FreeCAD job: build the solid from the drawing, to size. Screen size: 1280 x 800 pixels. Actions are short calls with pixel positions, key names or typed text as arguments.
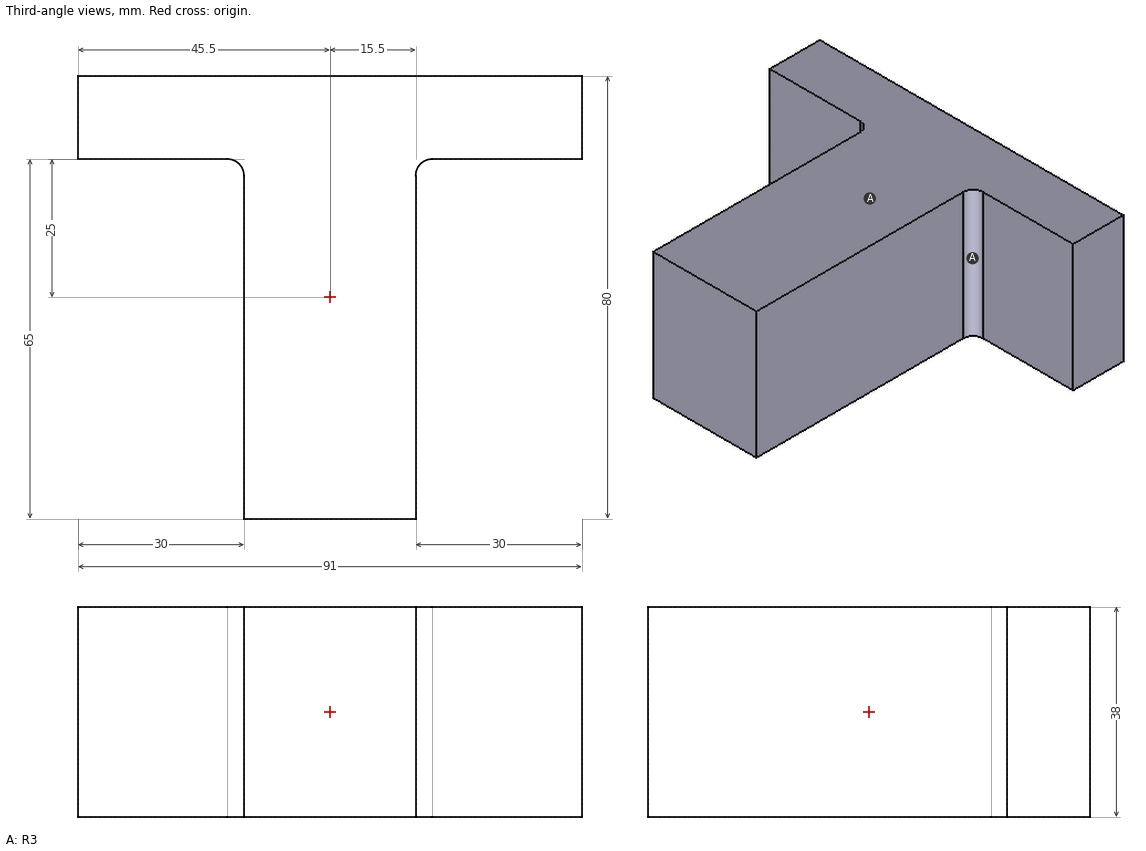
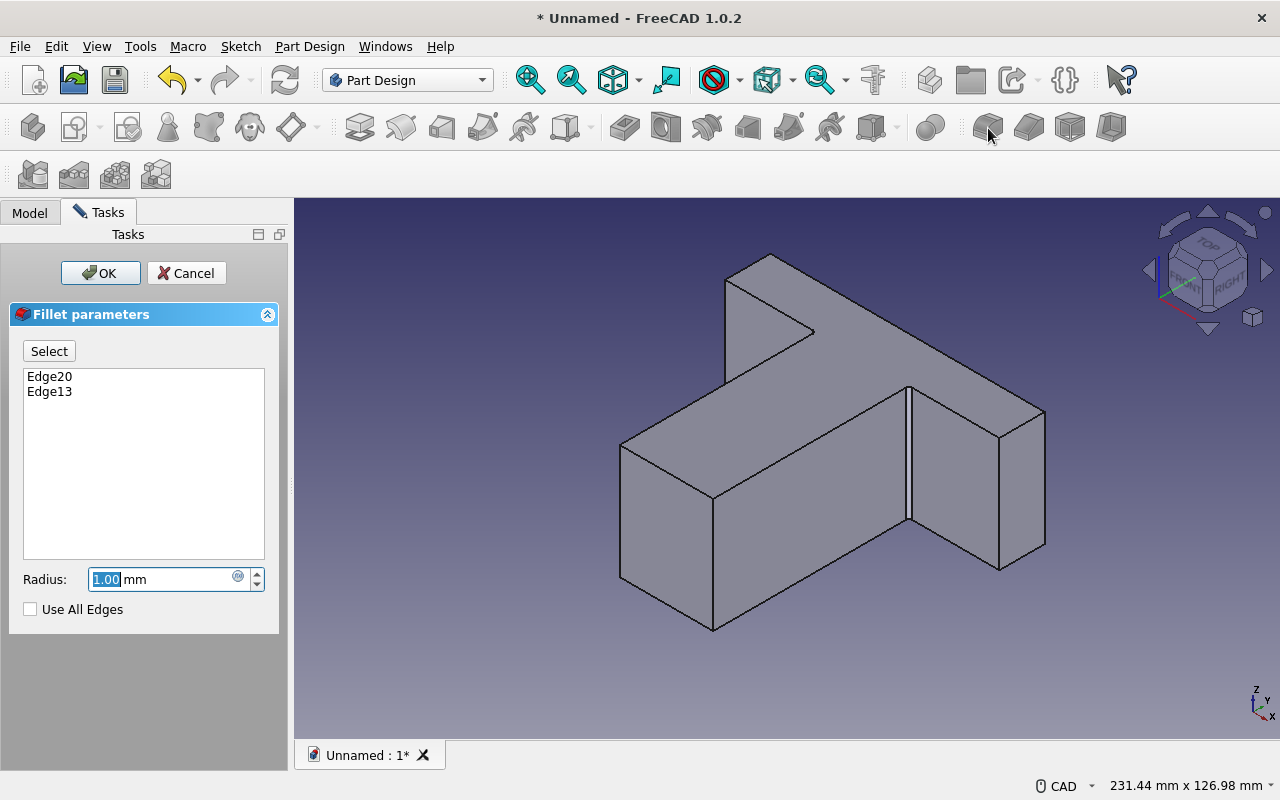
text(3)
key(Tab)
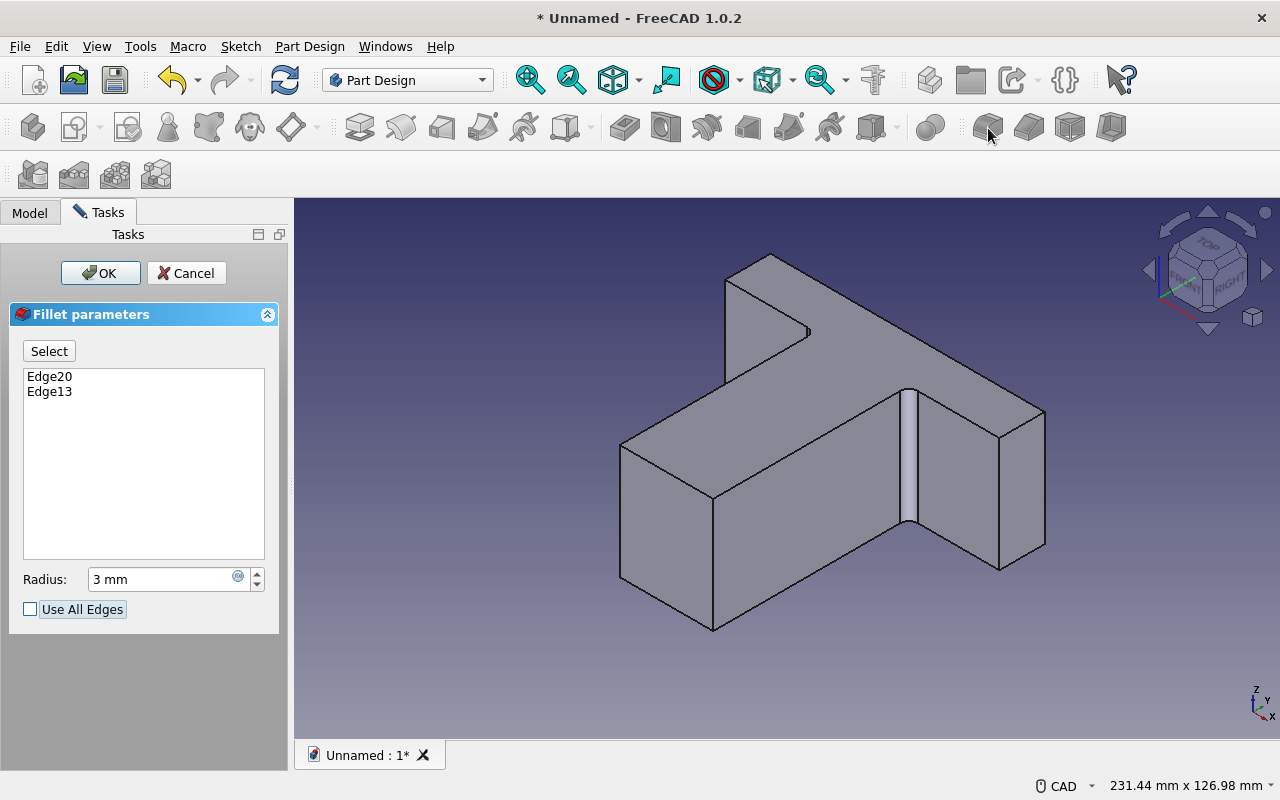
click(101, 273)